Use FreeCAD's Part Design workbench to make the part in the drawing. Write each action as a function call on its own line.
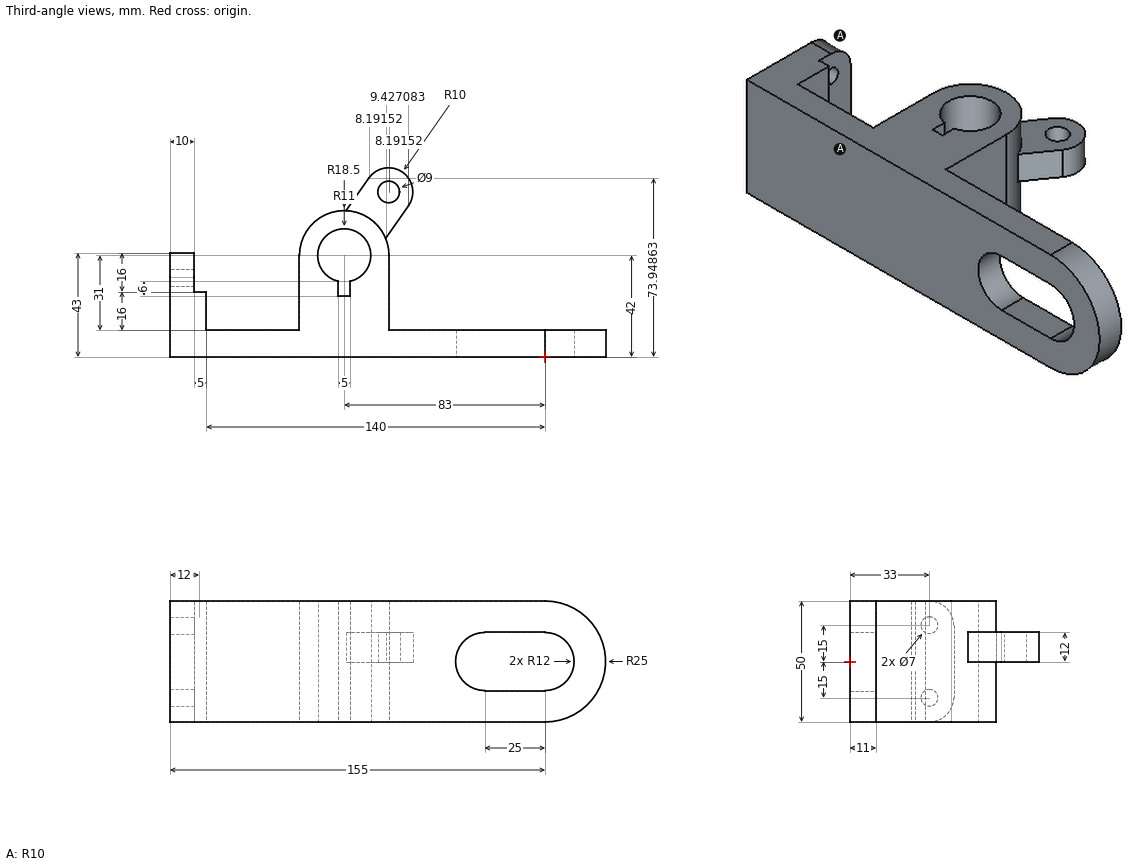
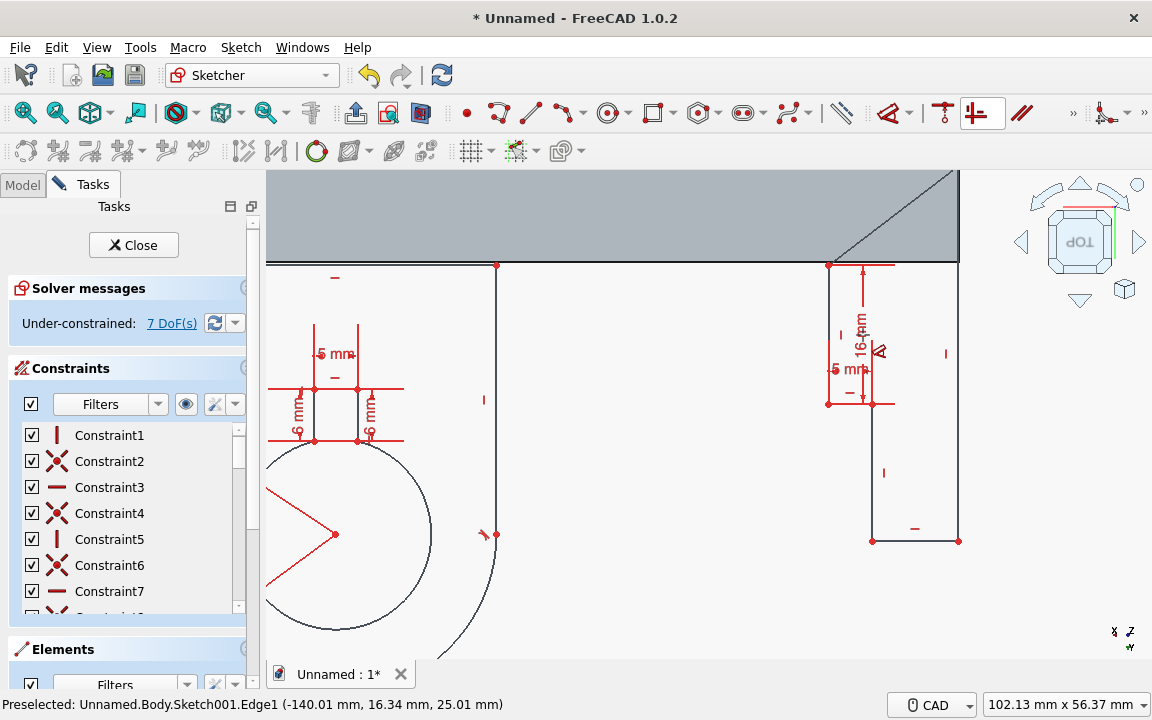
click(872, 445)
click(906, 473)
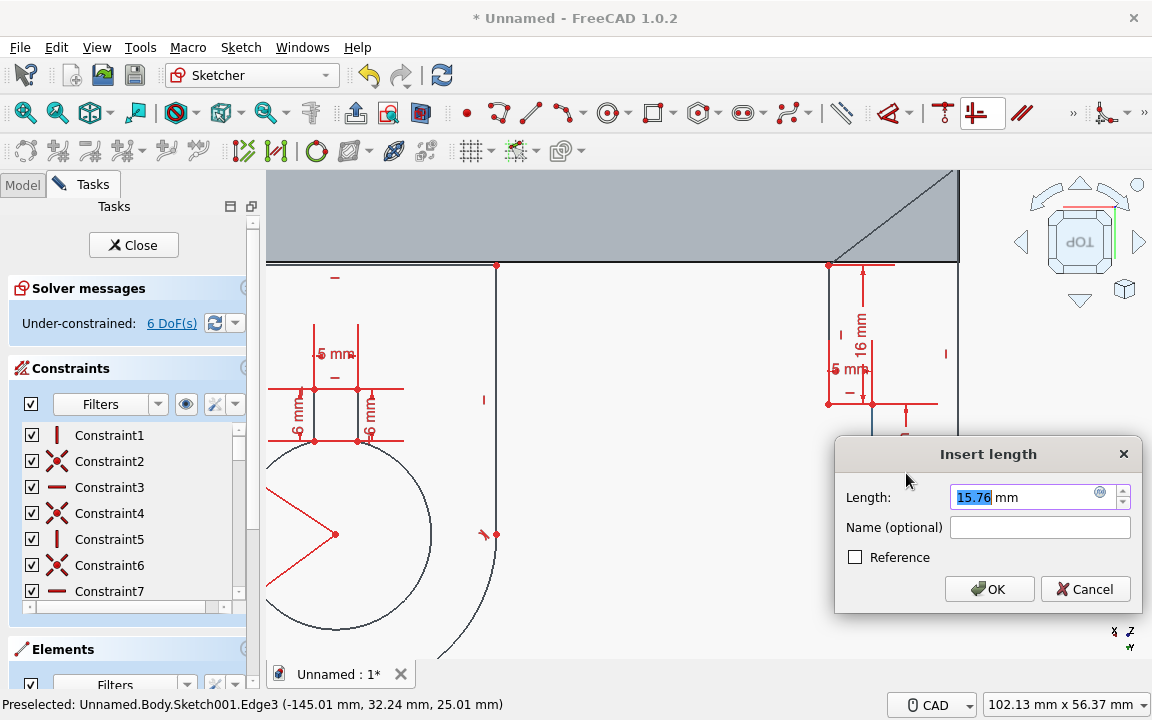
text(16)
key(Return)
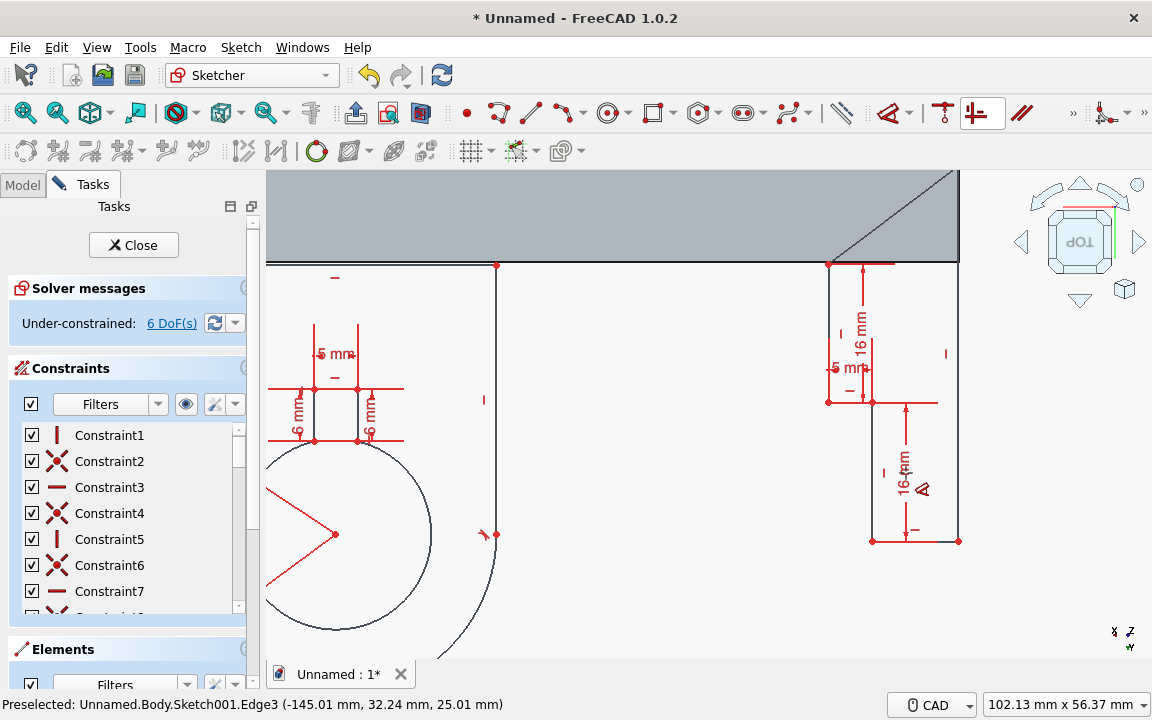
click(898, 542)
click(915, 576)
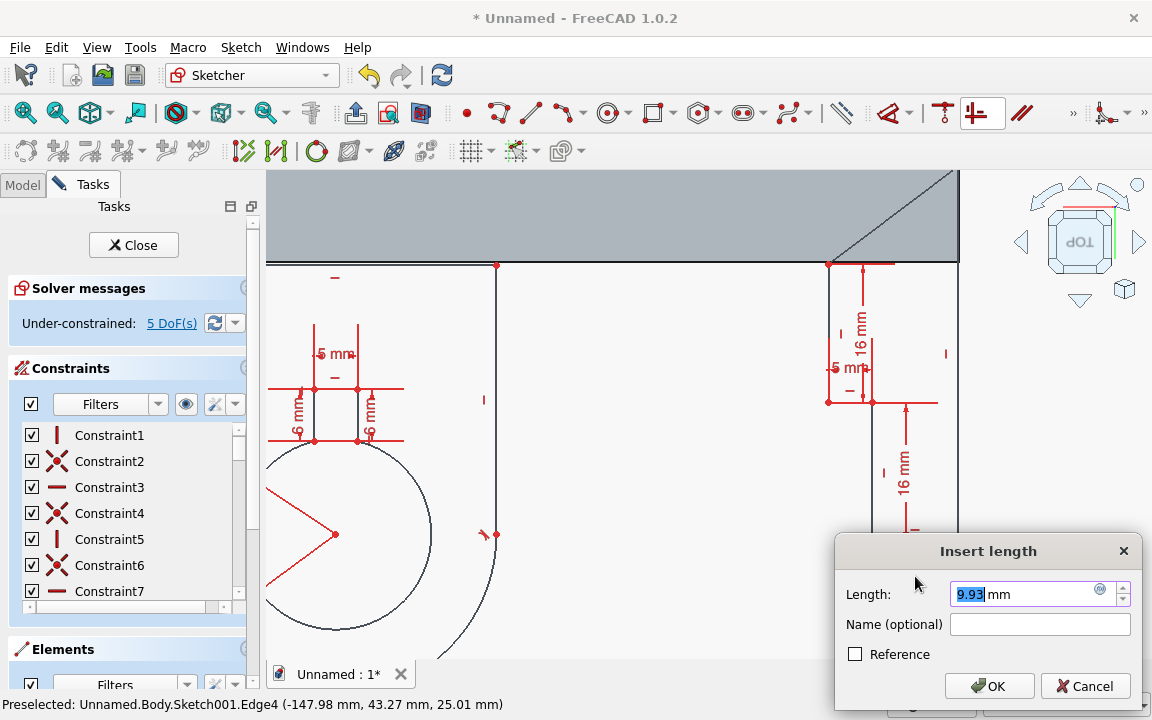
text(10)
key(Return)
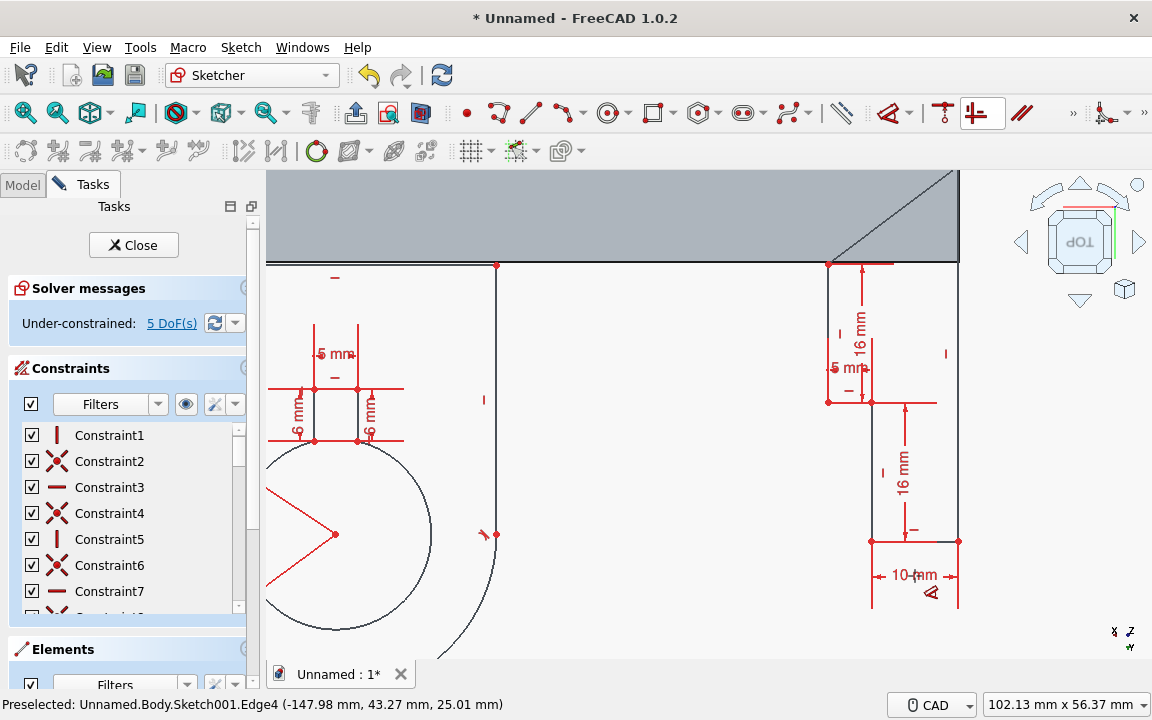
click(958, 429)
click(924, 370)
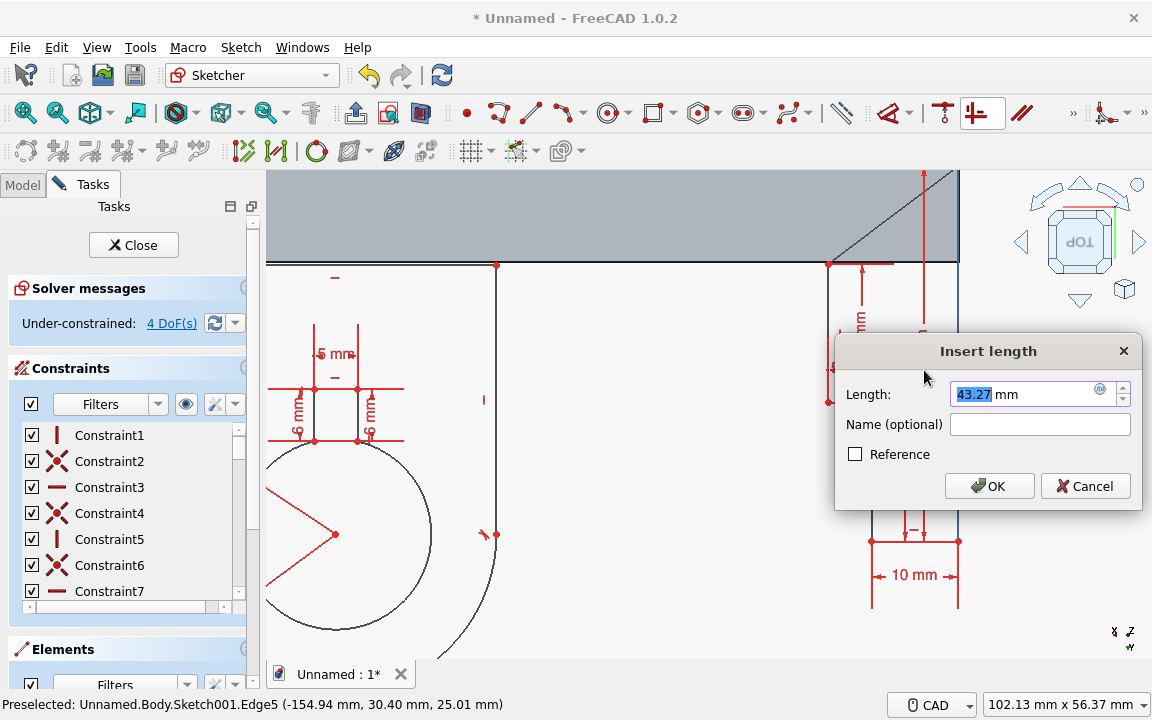
text(43)
key(Return)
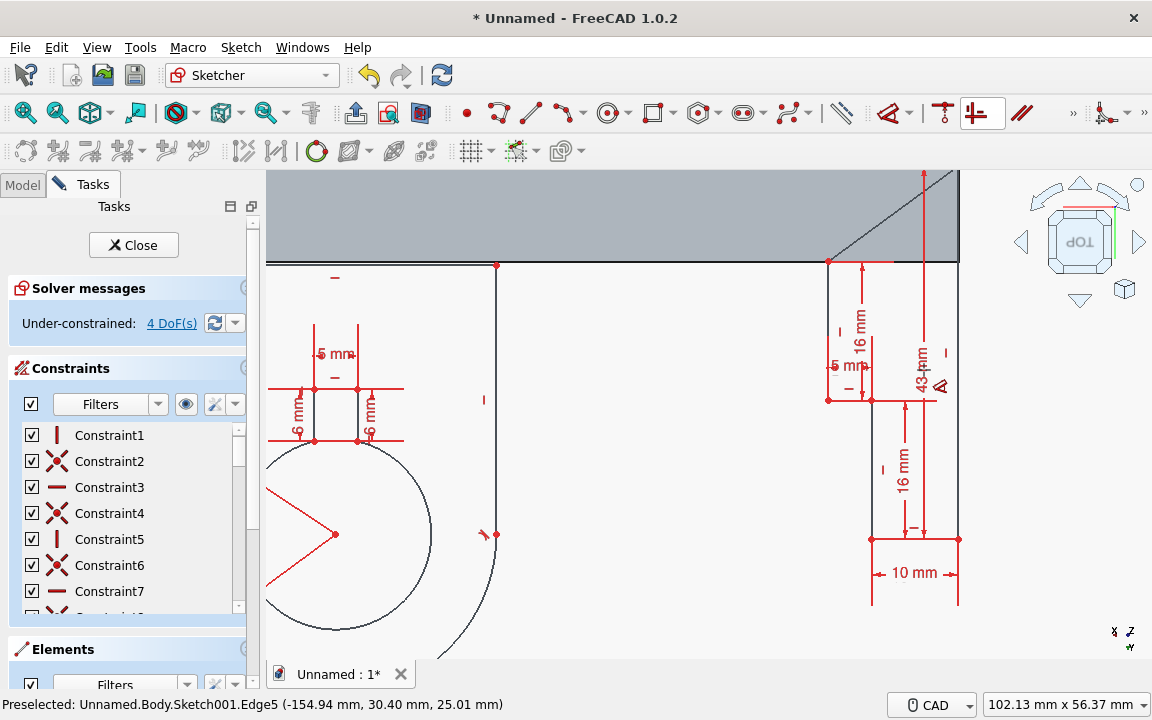
click(496, 454)
click(530, 400)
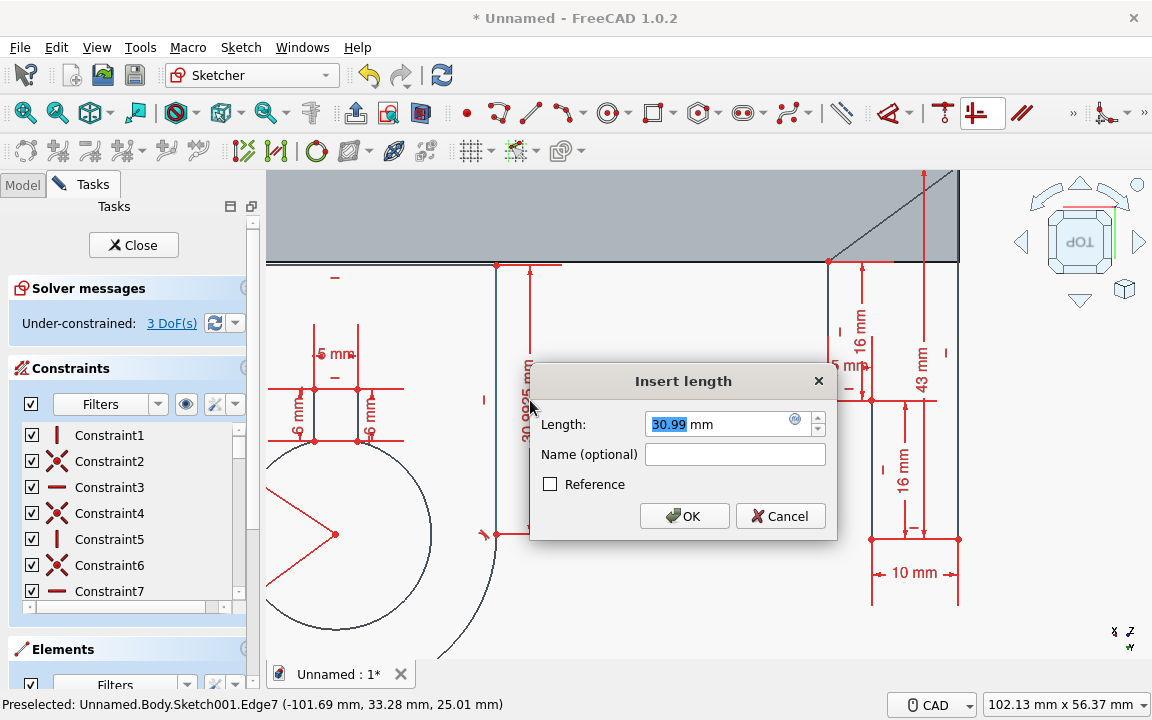
text(31)
key(Return)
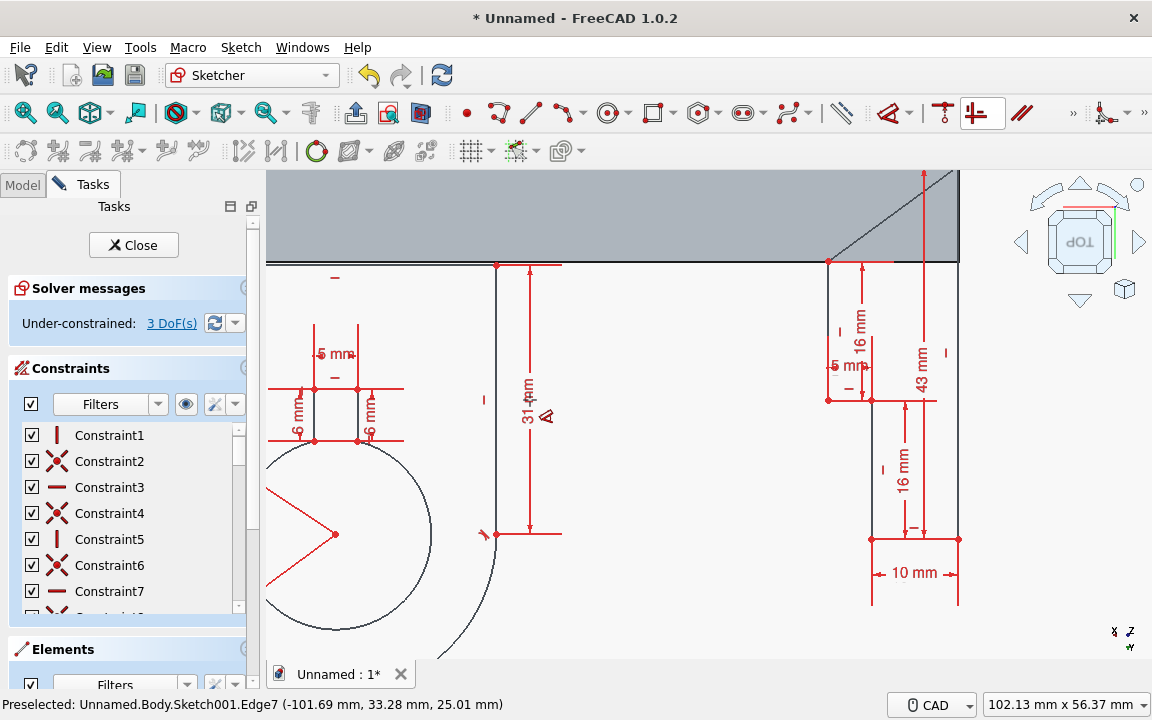
click(496, 534)
click(530, 366)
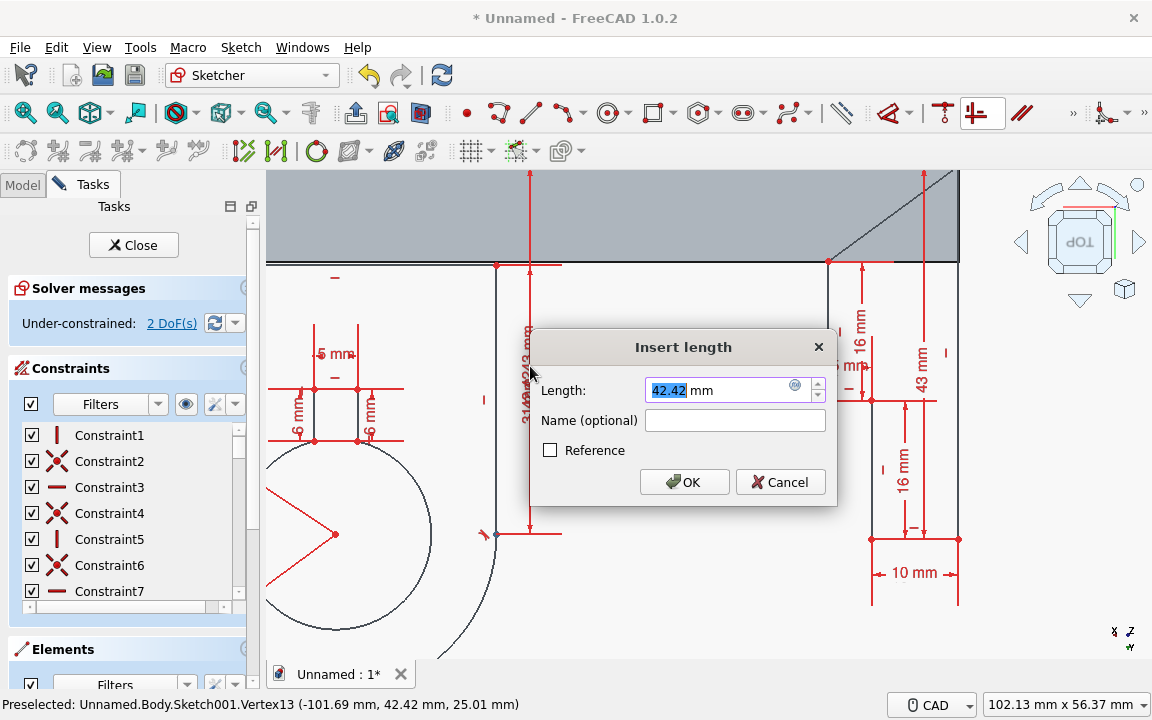
text(42)
key(Return)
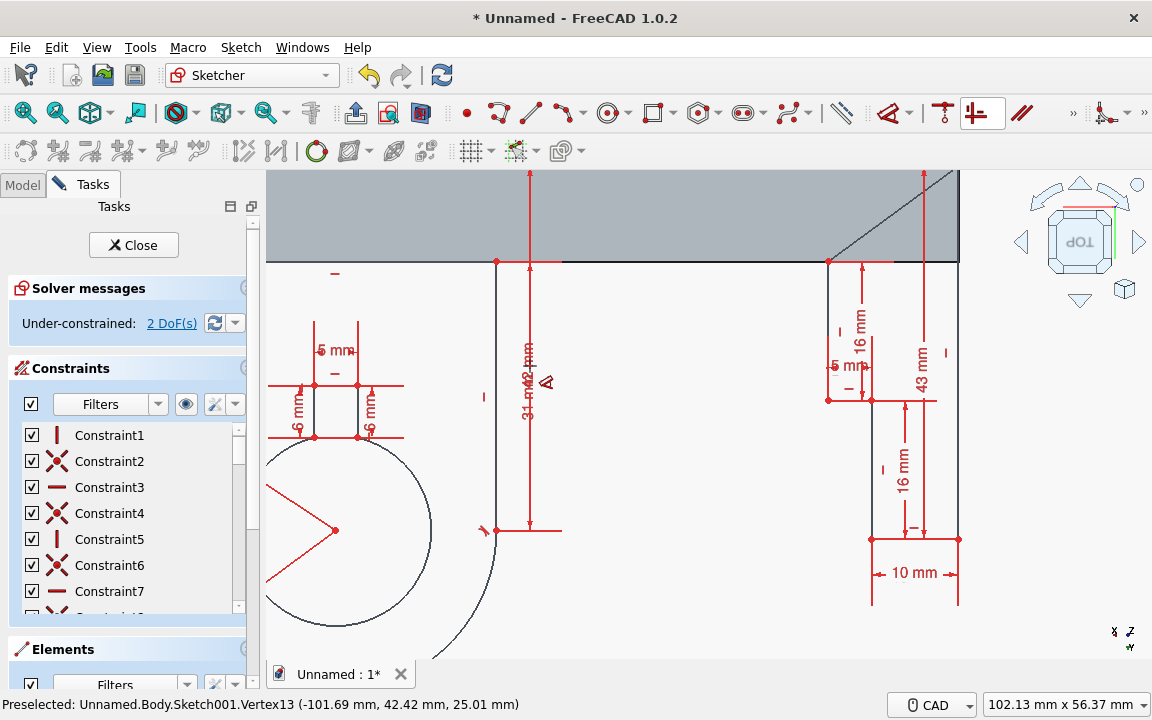
click(336, 531)
click(315, 565)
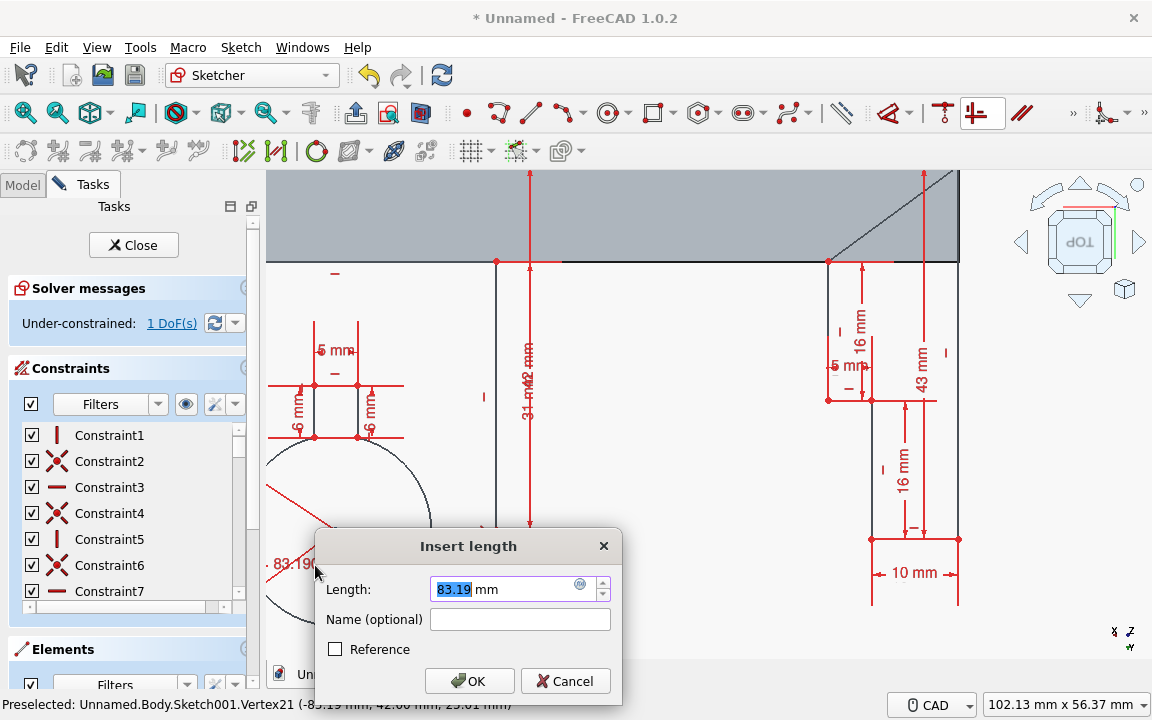
text(83)
key(Return)